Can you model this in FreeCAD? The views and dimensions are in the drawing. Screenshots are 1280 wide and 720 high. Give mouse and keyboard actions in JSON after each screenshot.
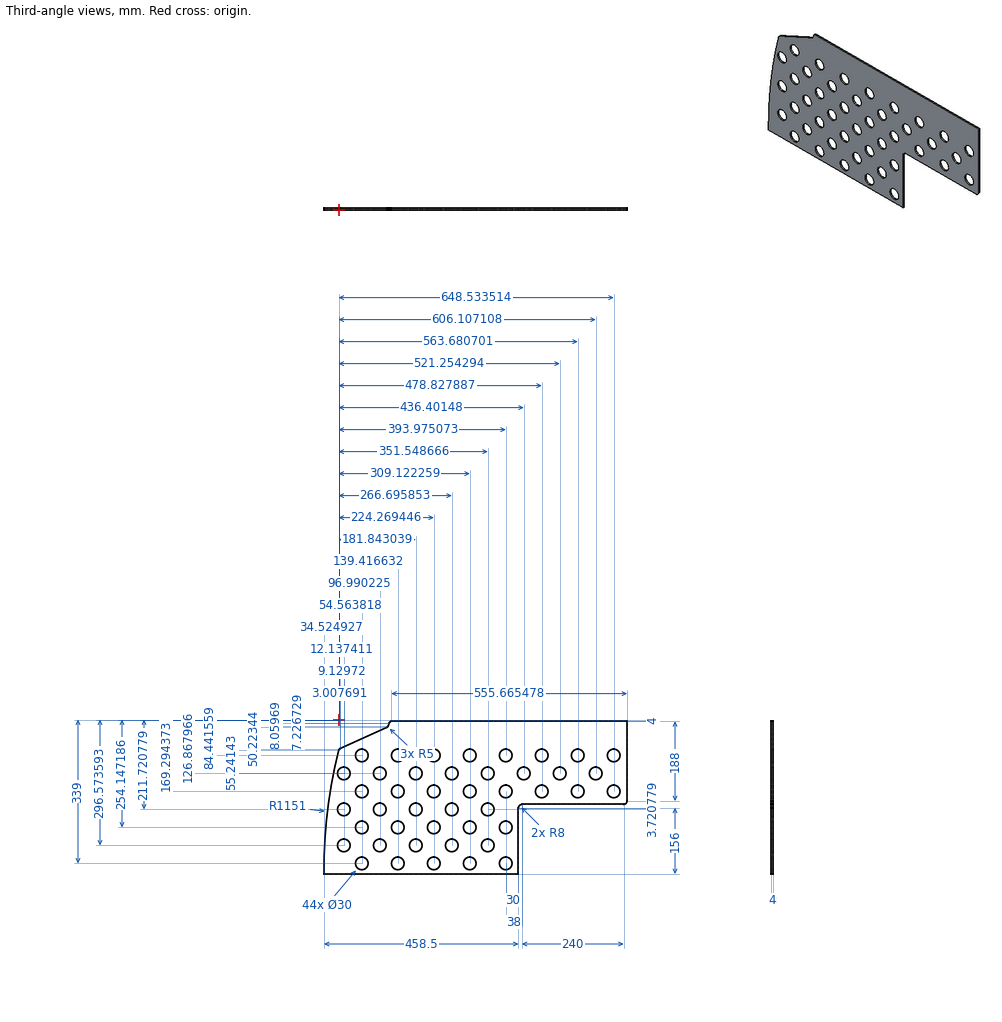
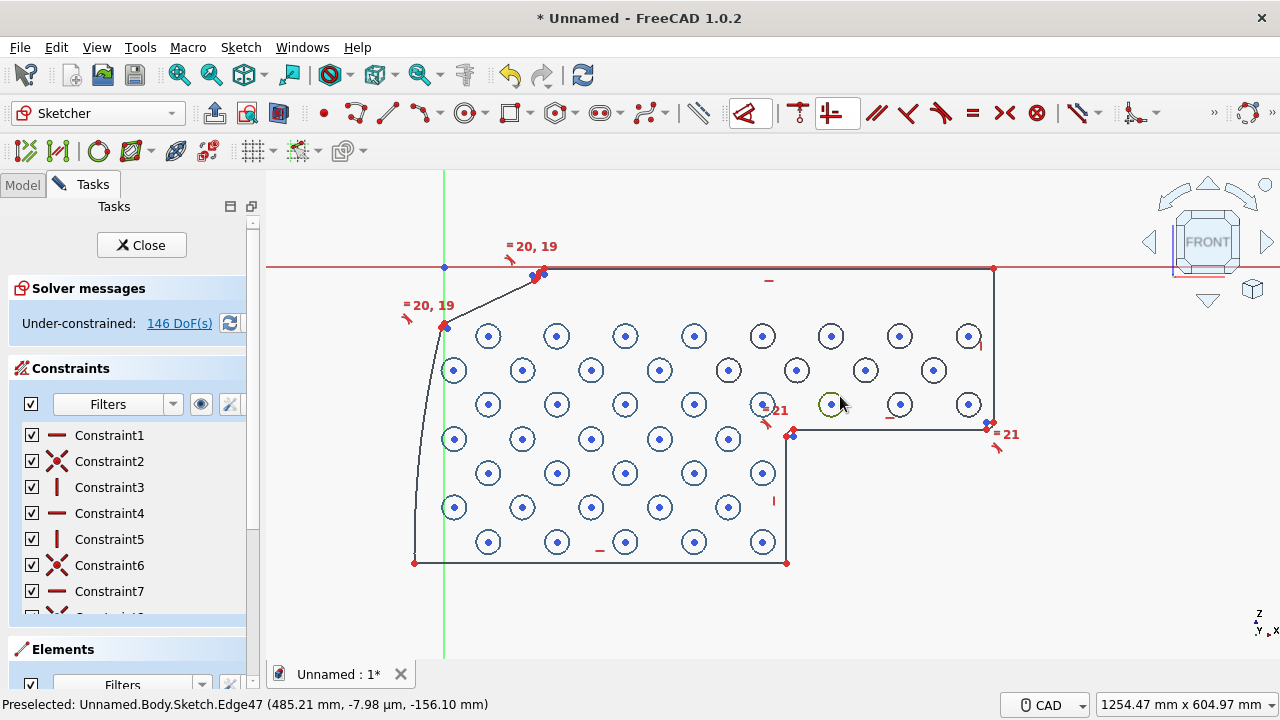
{"action": "left_click", "coordinate": [909, 396]}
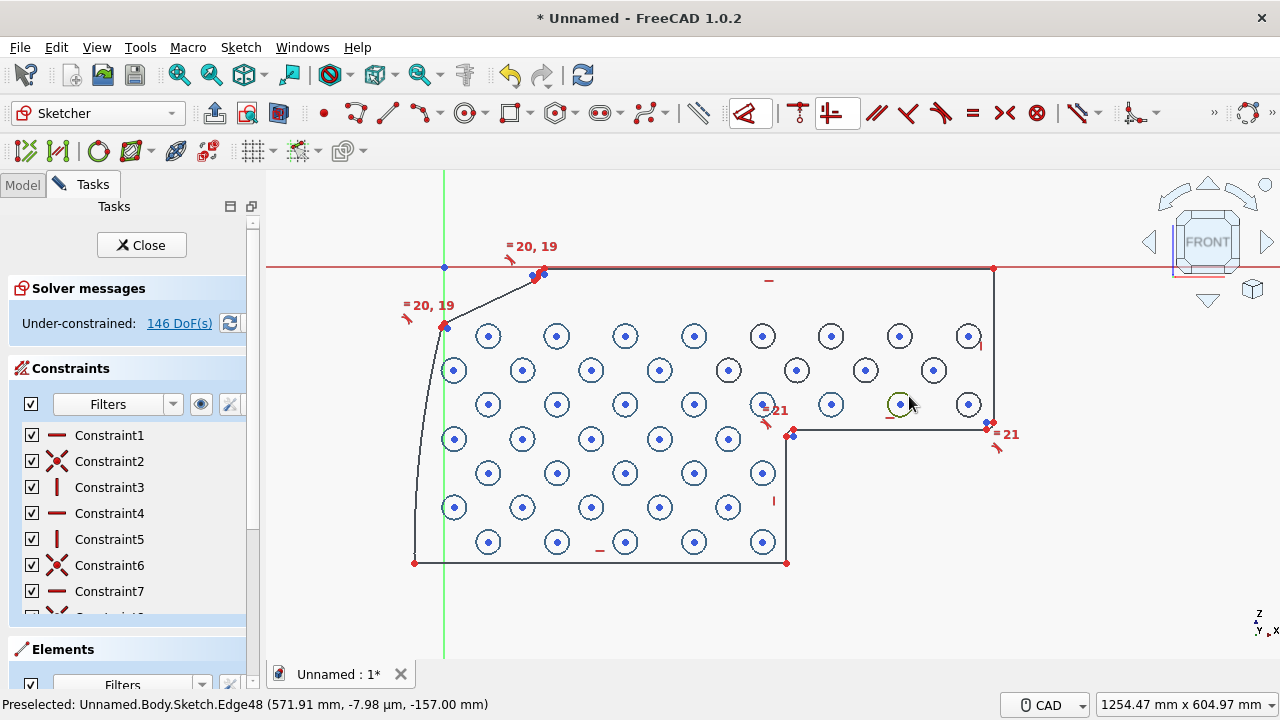
{"action": "left_click", "coordinate": [977, 396]}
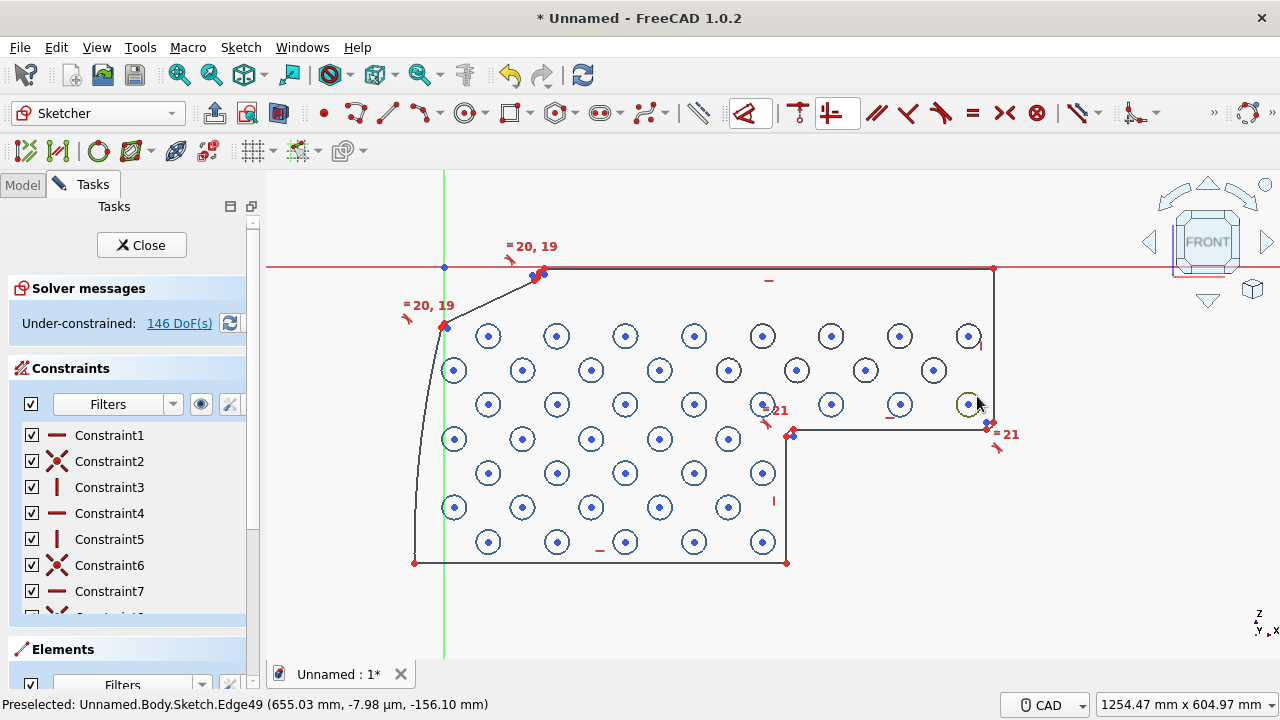
{"action": "left_click", "coordinate": [737, 362]}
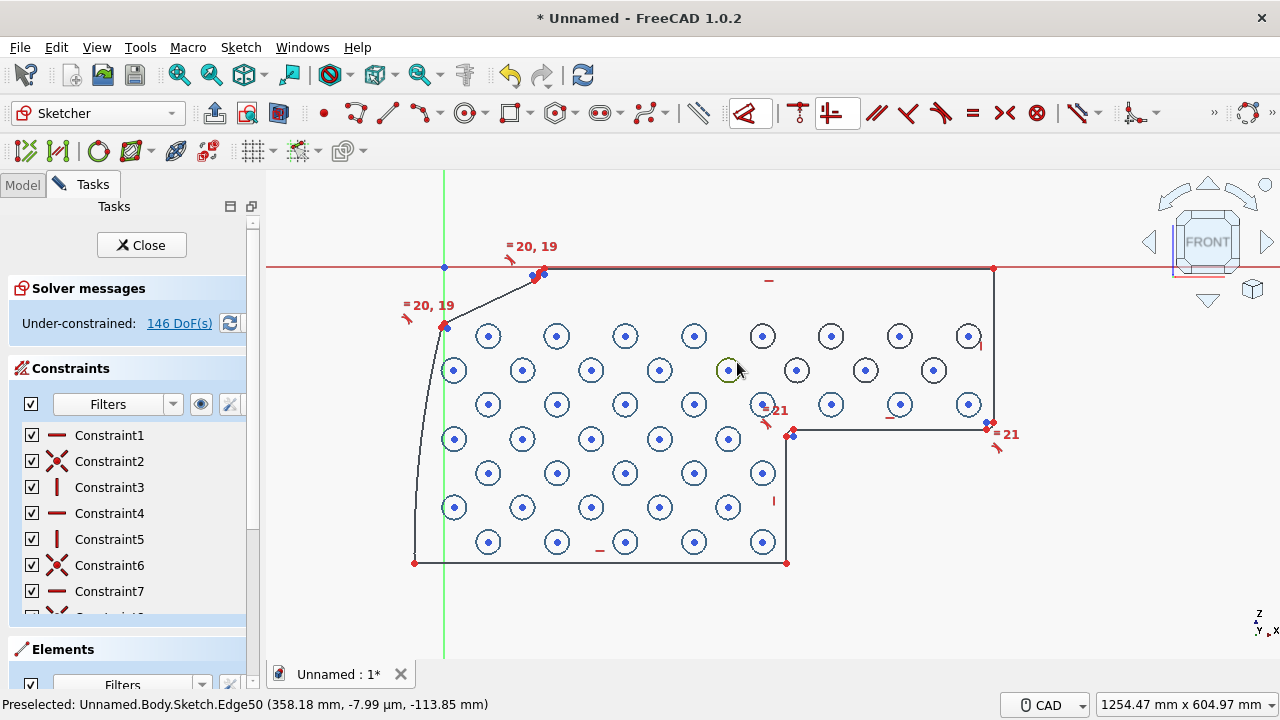
{"action": "left_click", "coordinate": [805, 362]}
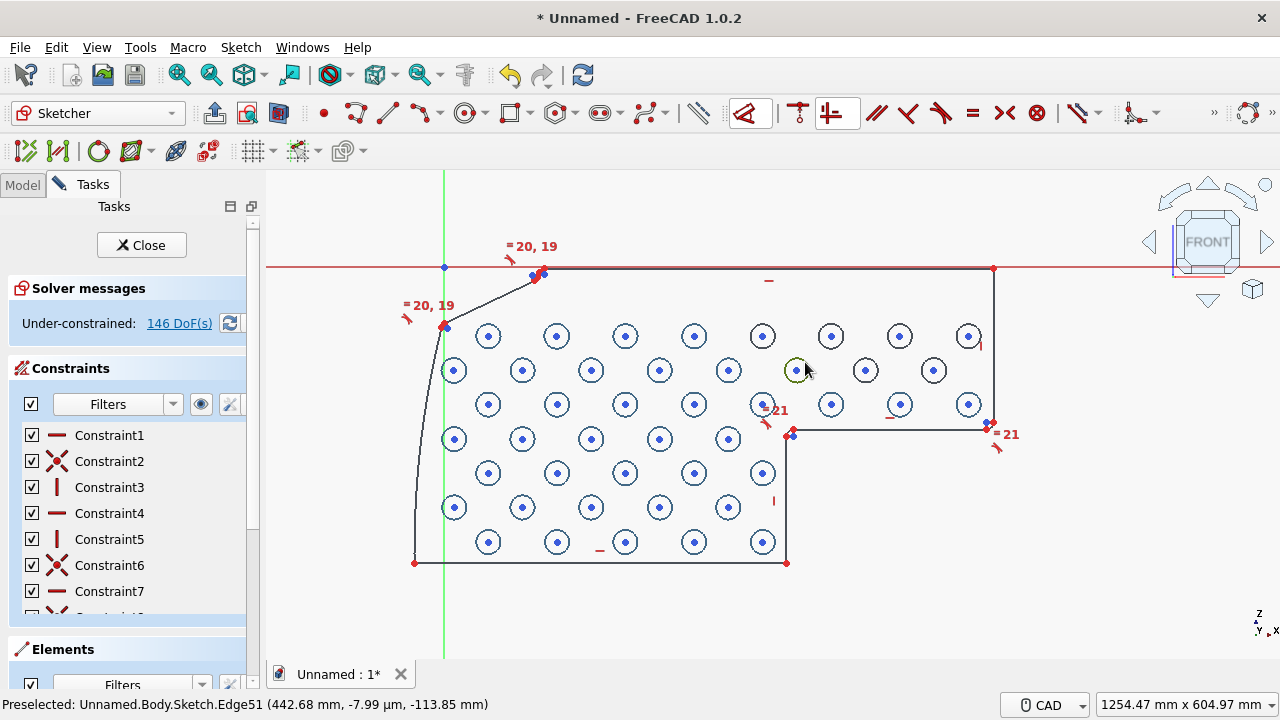
{"action": "left_click", "coordinate": [771, 328]}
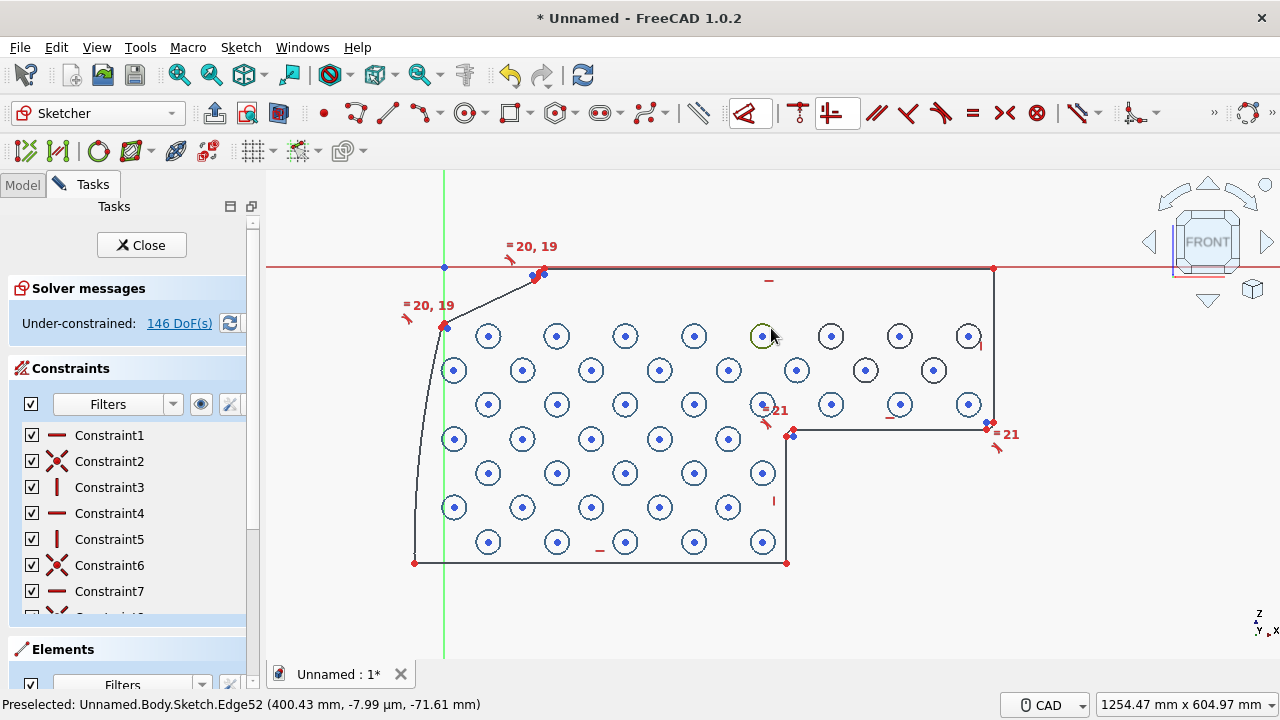
{"action": "left_click", "coordinate": [840, 327]}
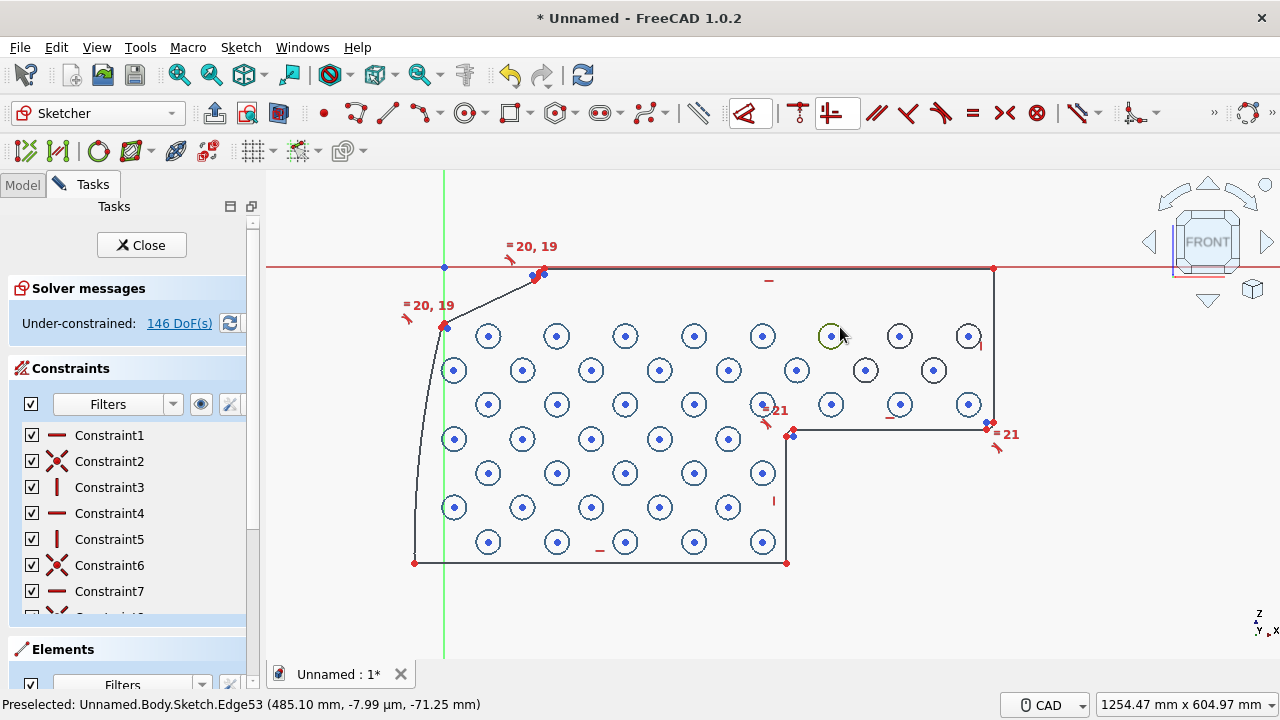
{"action": "left_click", "coordinate": [874, 362]}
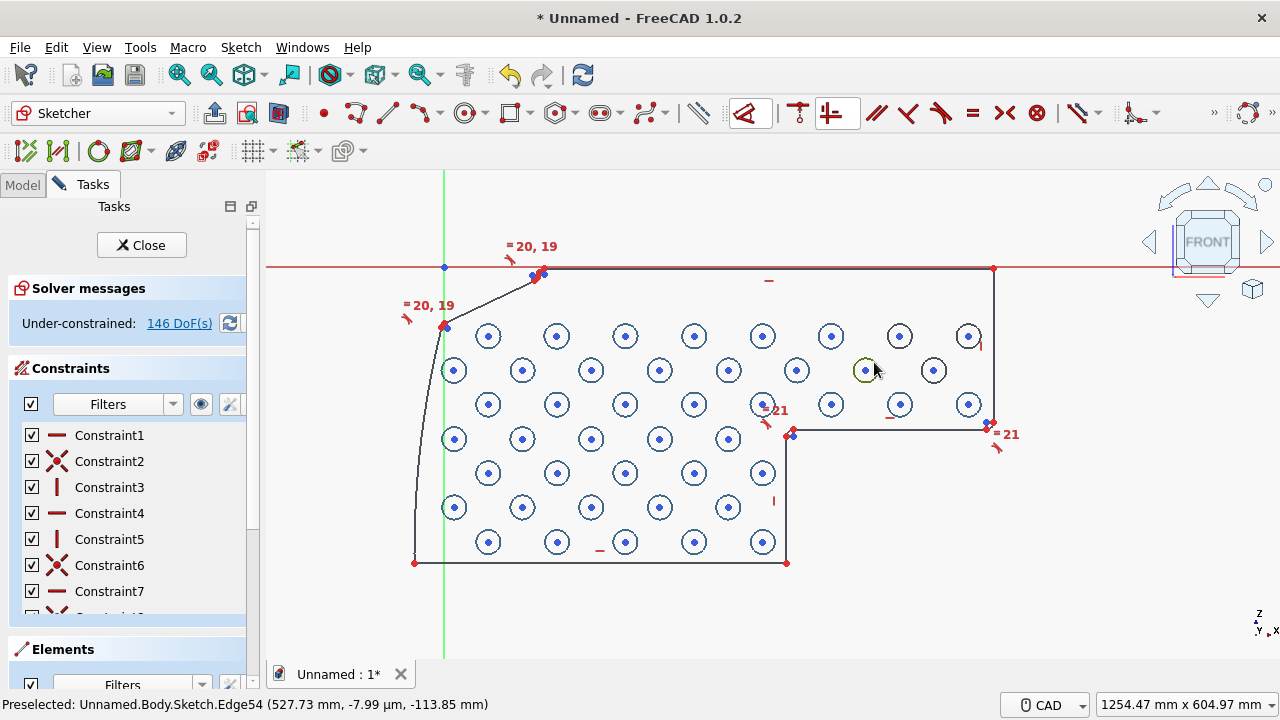
{"action": "left_click", "coordinate": [943, 362]}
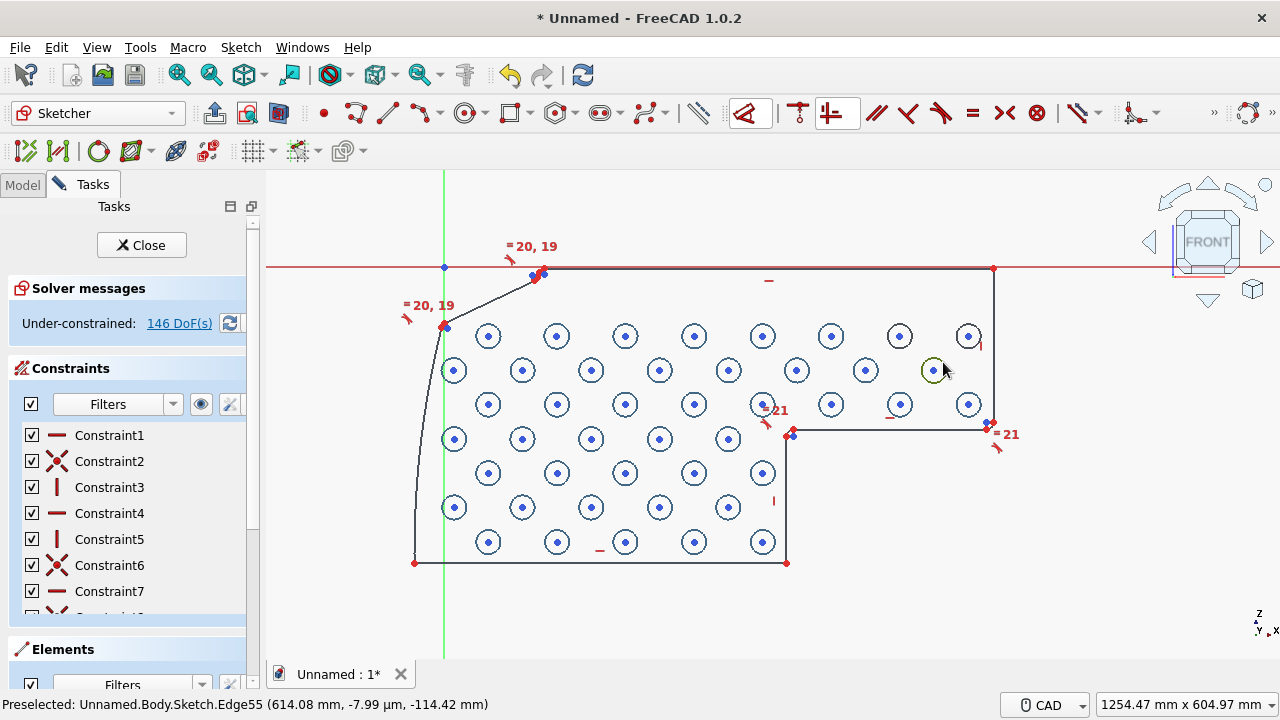
{"action": "left_click", "coordinate": [908, 328]}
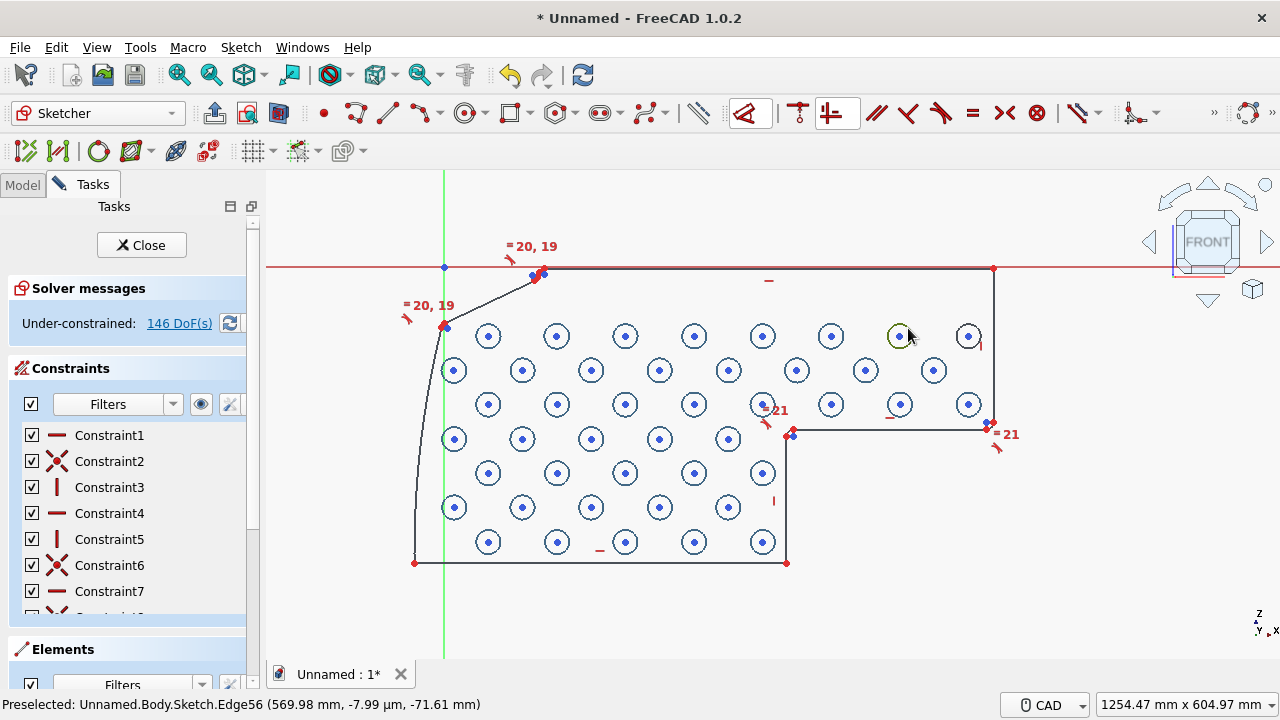
{"action": "left_click", "coordinate": [977, 328]}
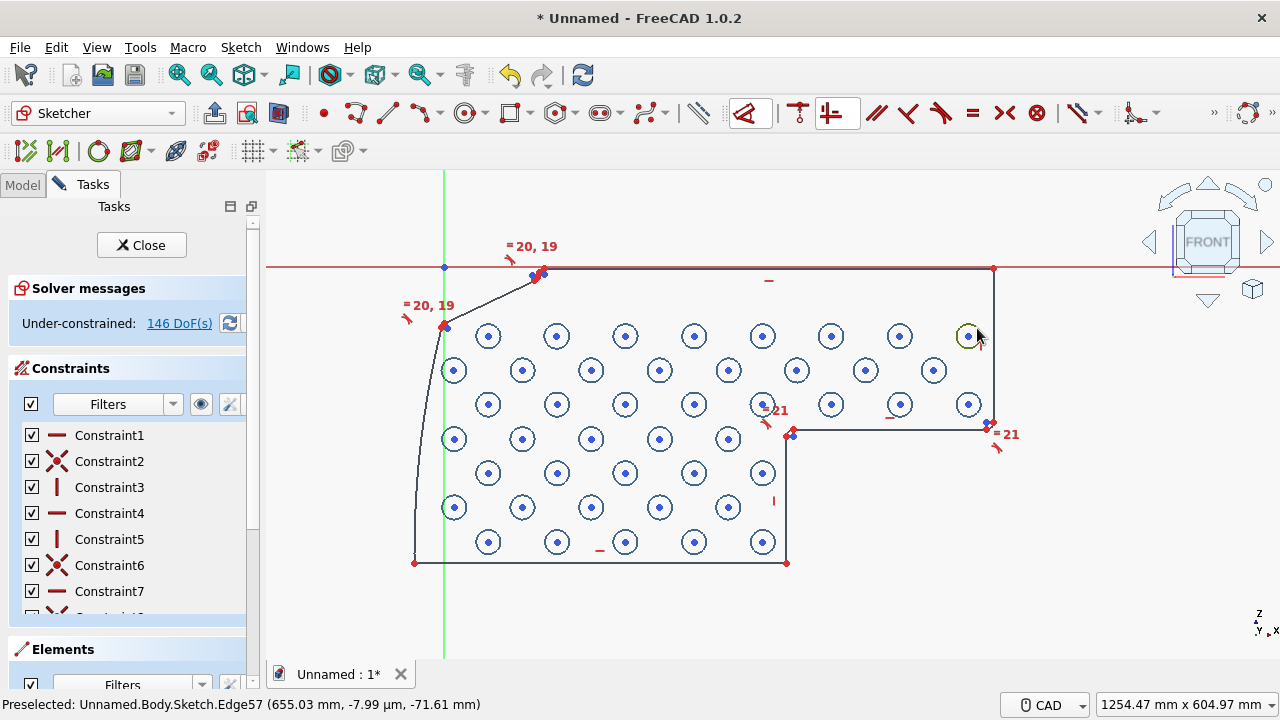
{"action": "left_click", "coordinate": [974, 114]}